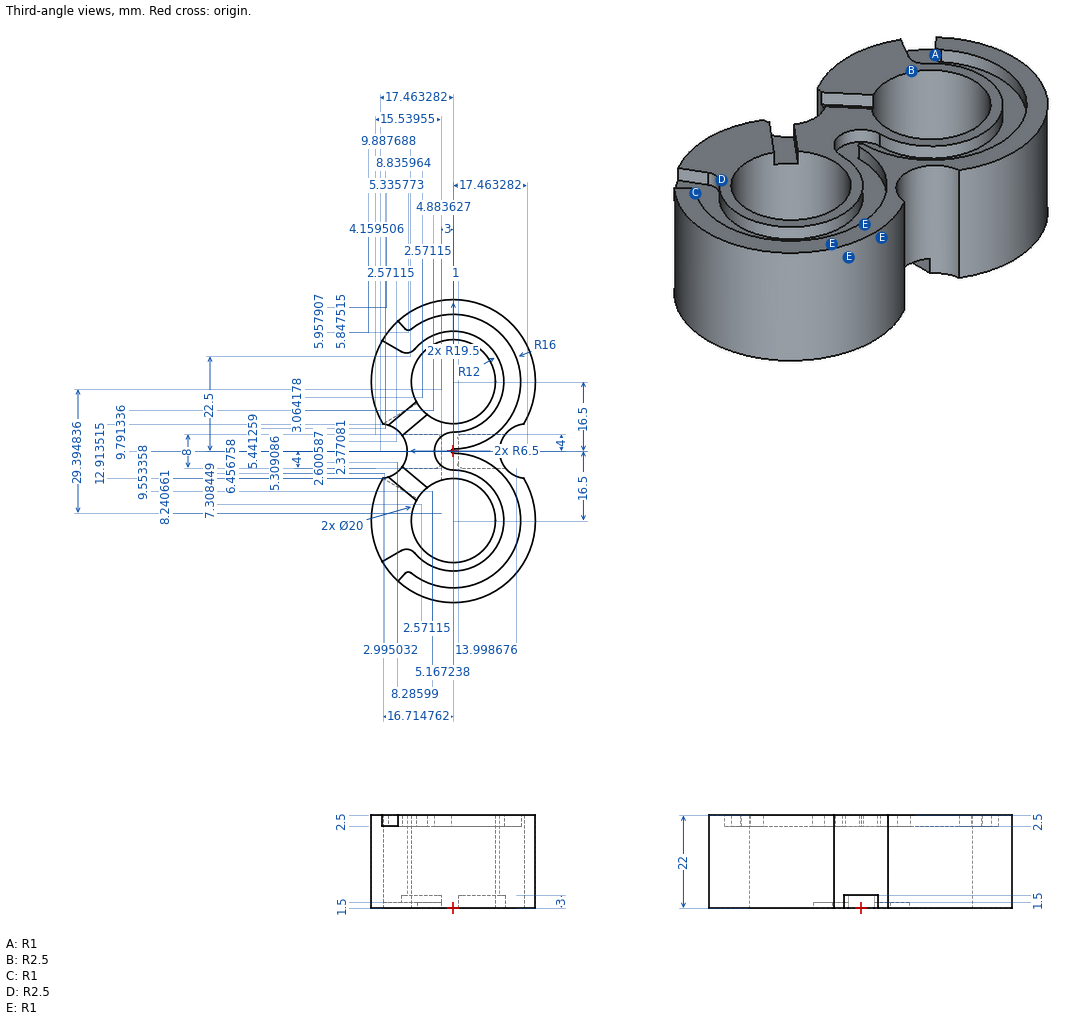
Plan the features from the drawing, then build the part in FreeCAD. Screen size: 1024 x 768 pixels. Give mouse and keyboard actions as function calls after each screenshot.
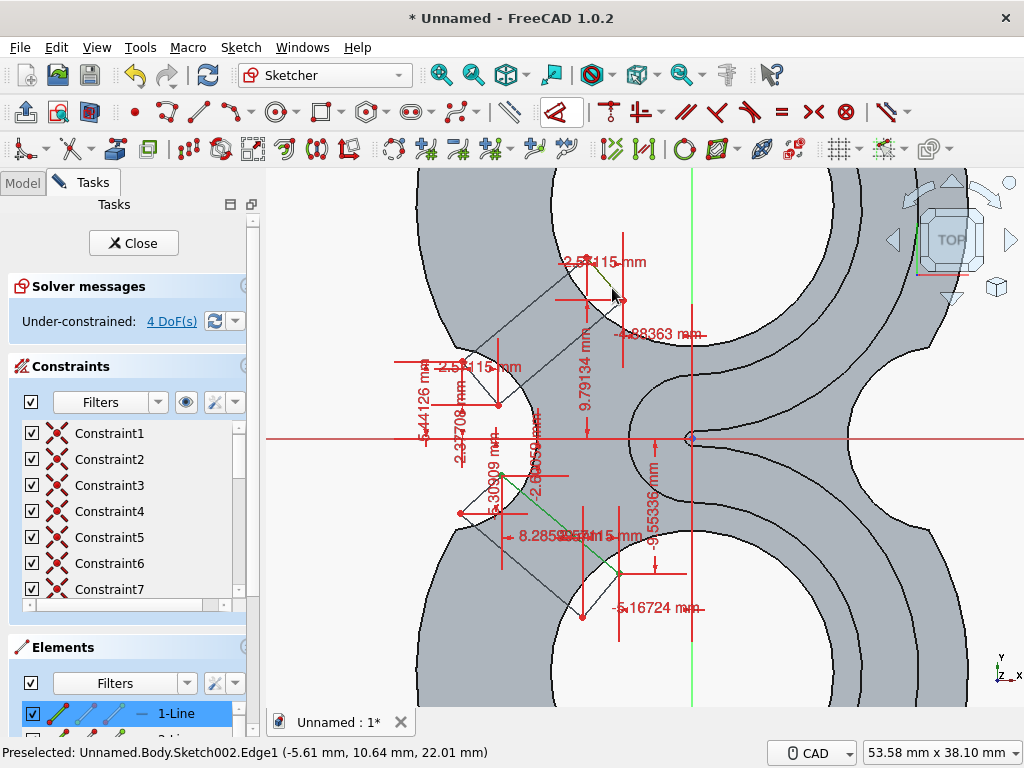
key(i)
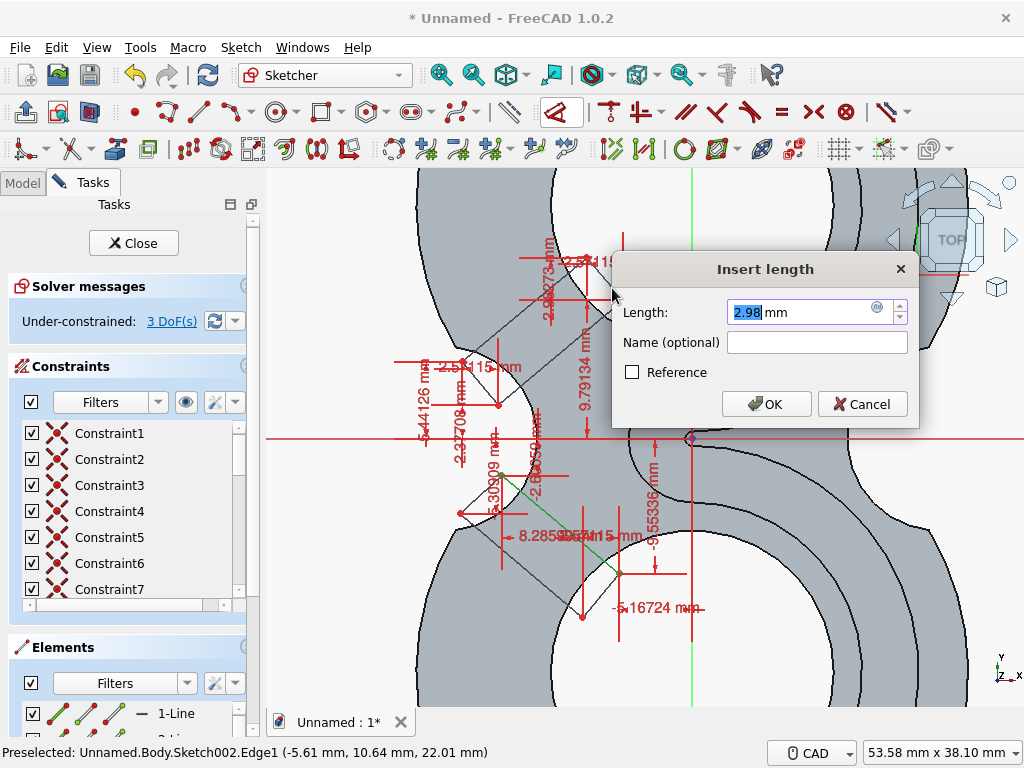
text(3.064178)
key(Return)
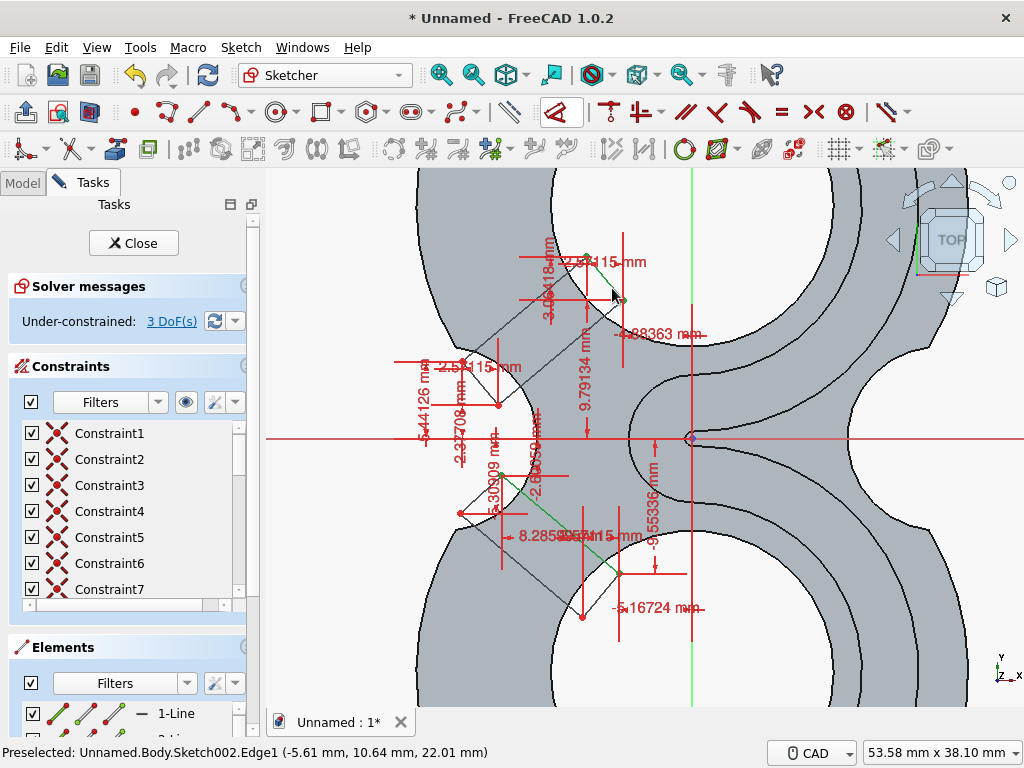
click(499, 330)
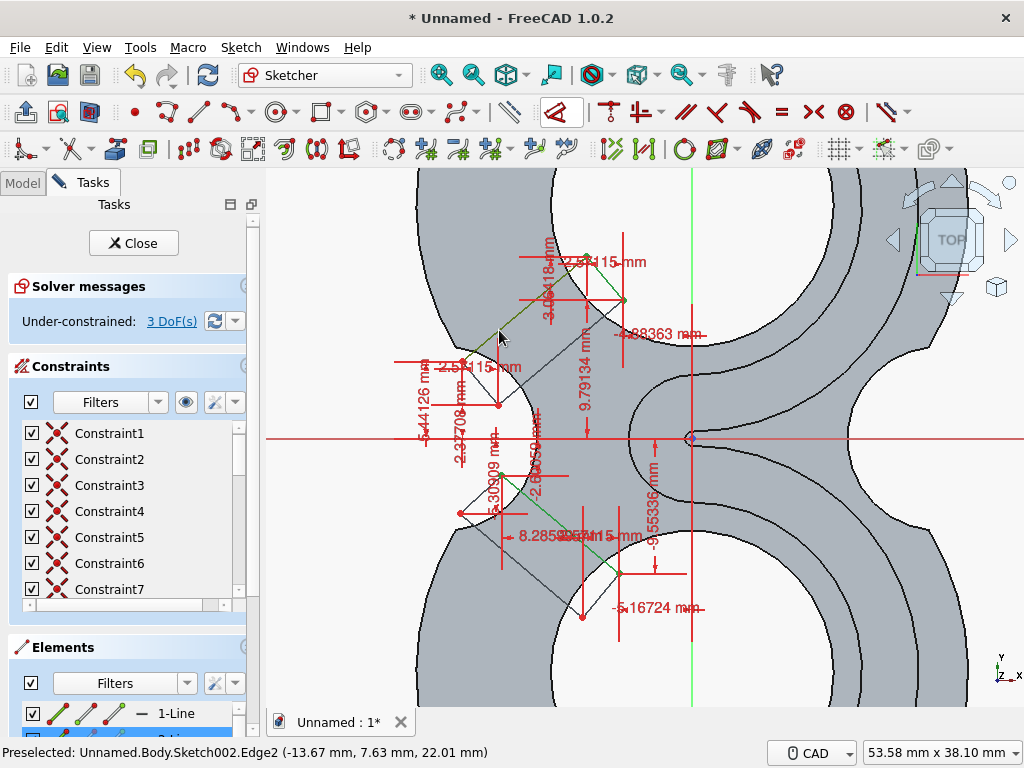
key(l)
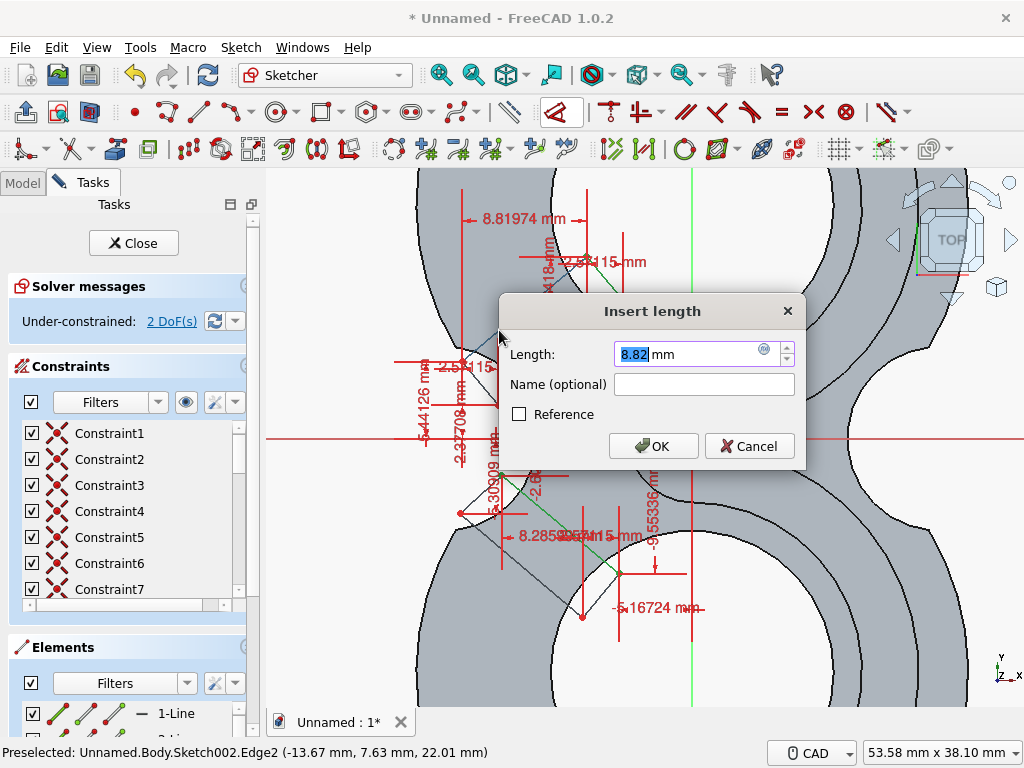
text(8.835964)
key(Return)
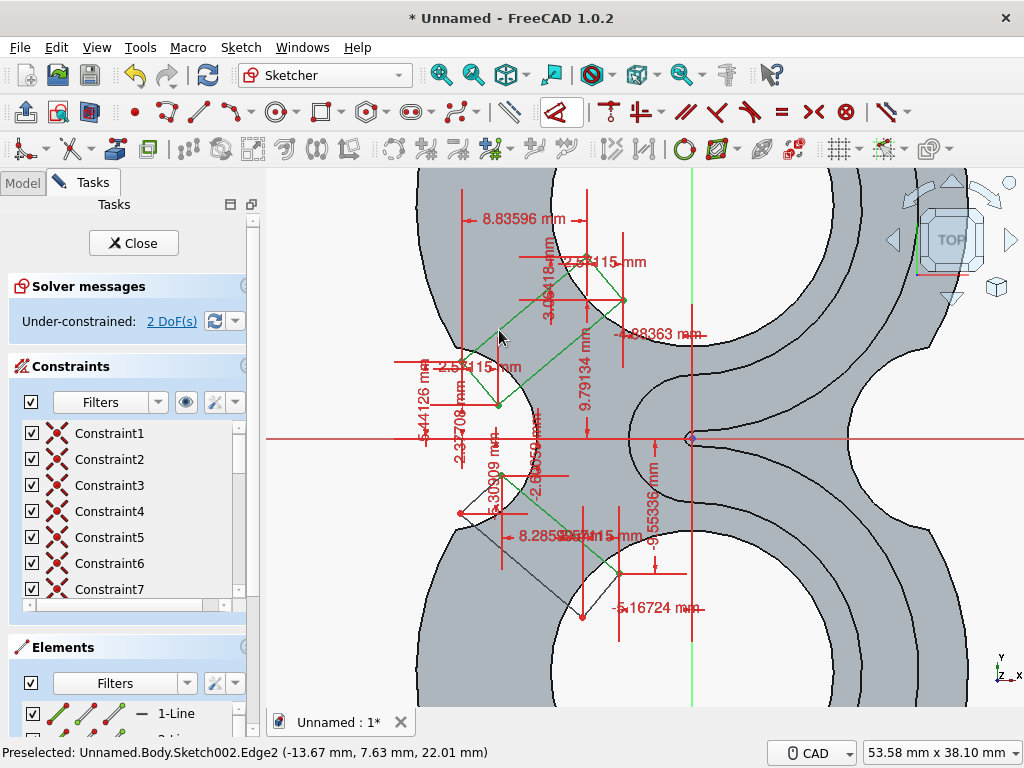
click(473, 502)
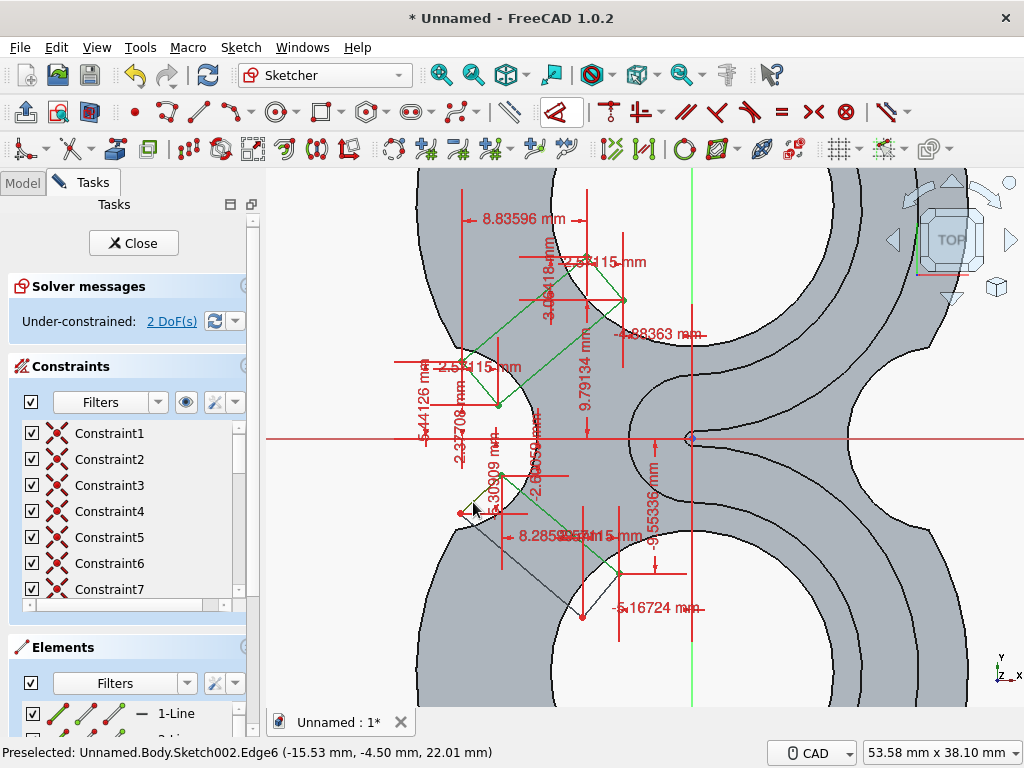
key(l)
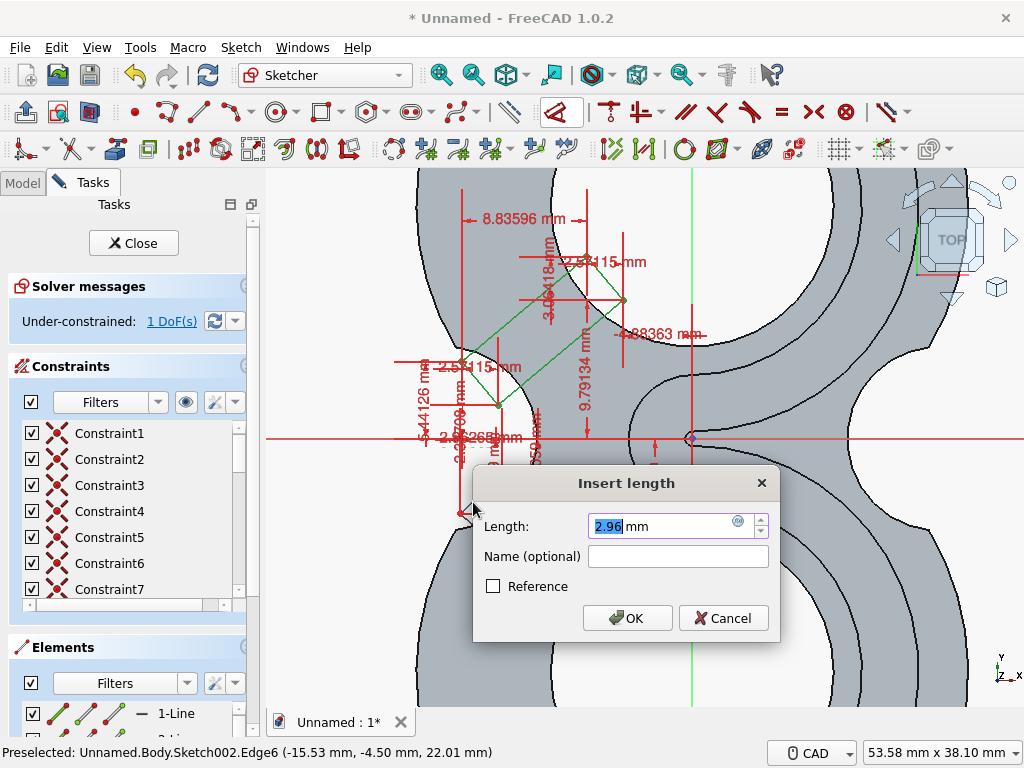
text(2.995032)
key(Return)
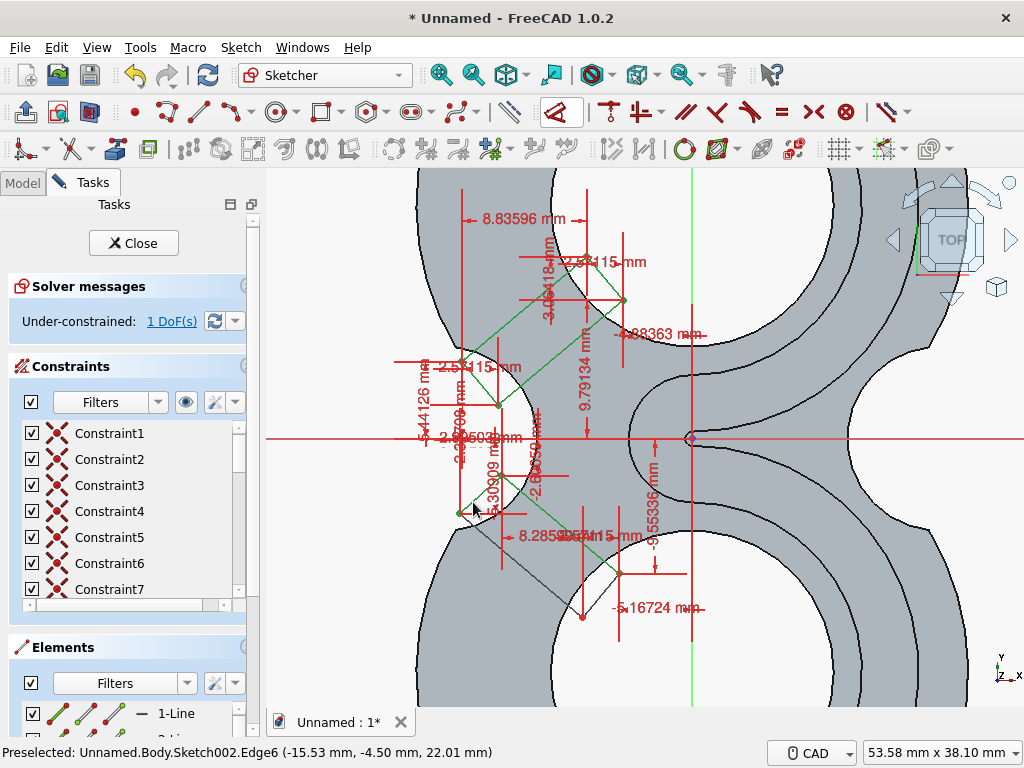
click(497, 545)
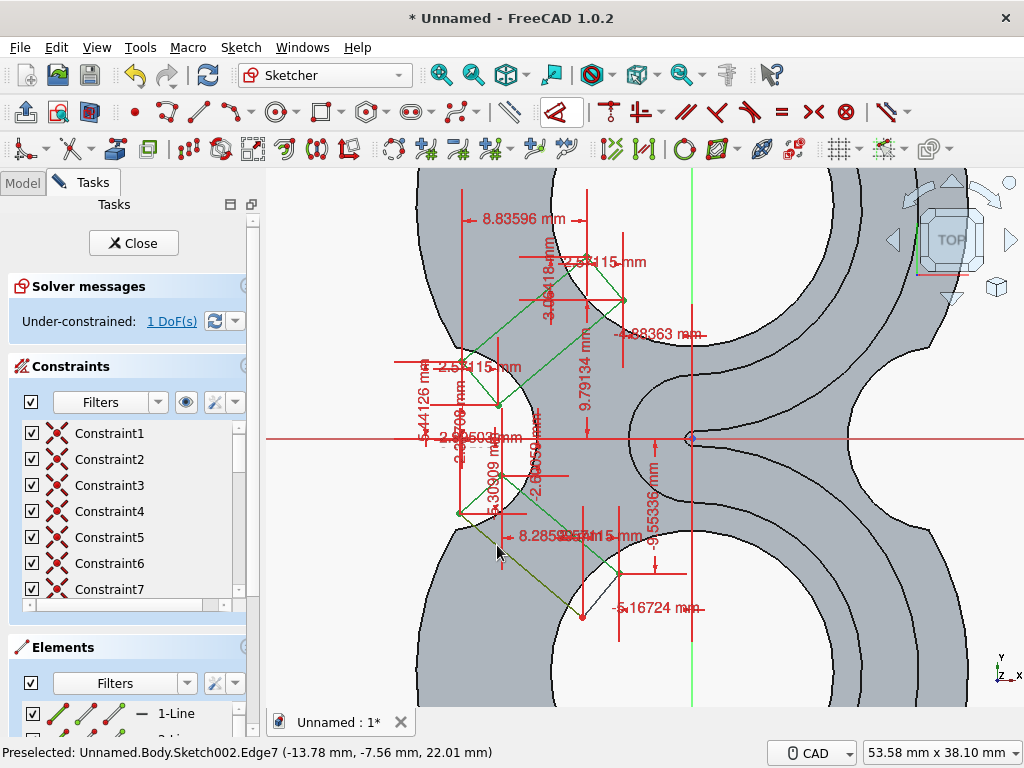
click(578, 112)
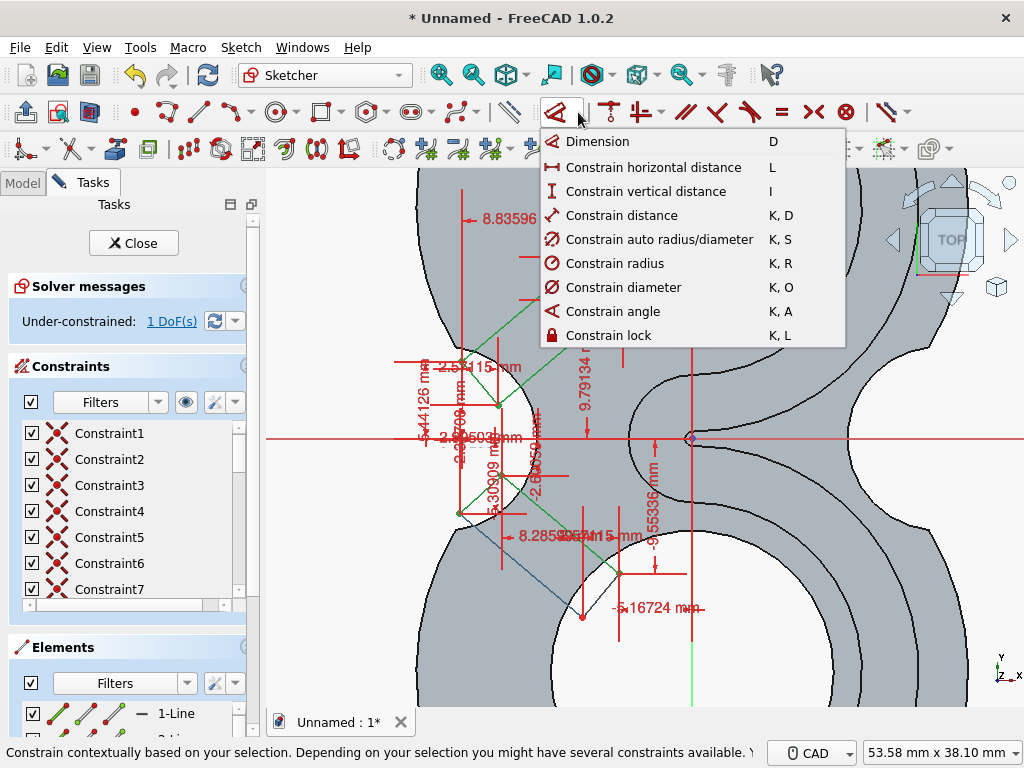
click(693, 191)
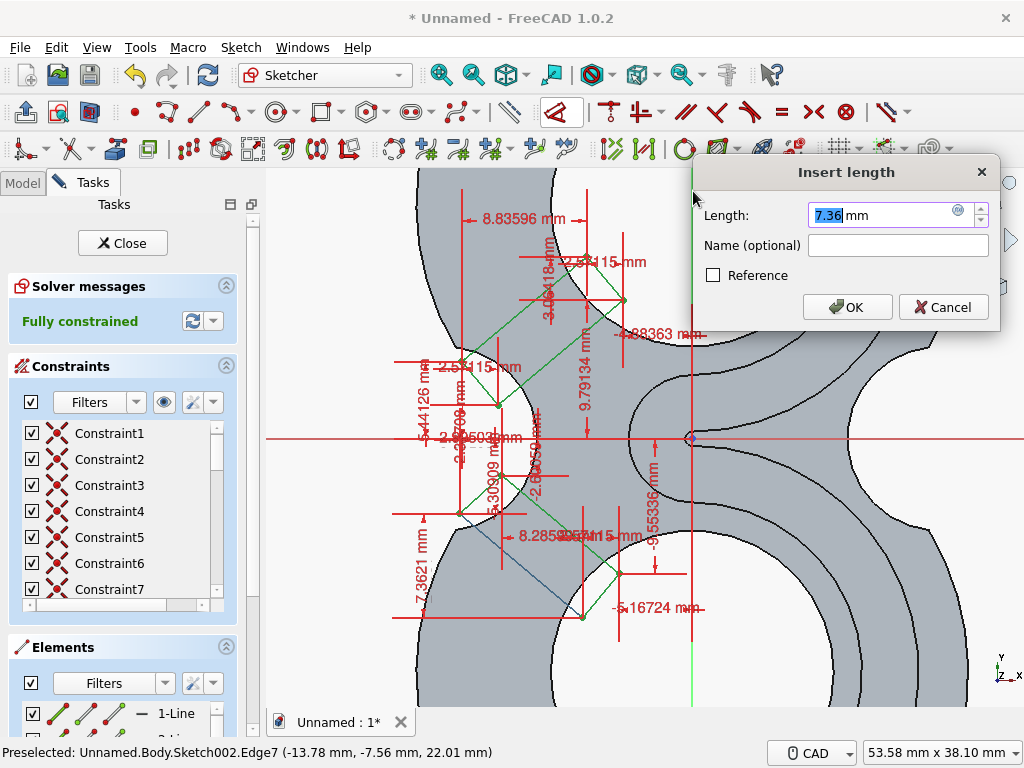
text(7.308449)
key(Return)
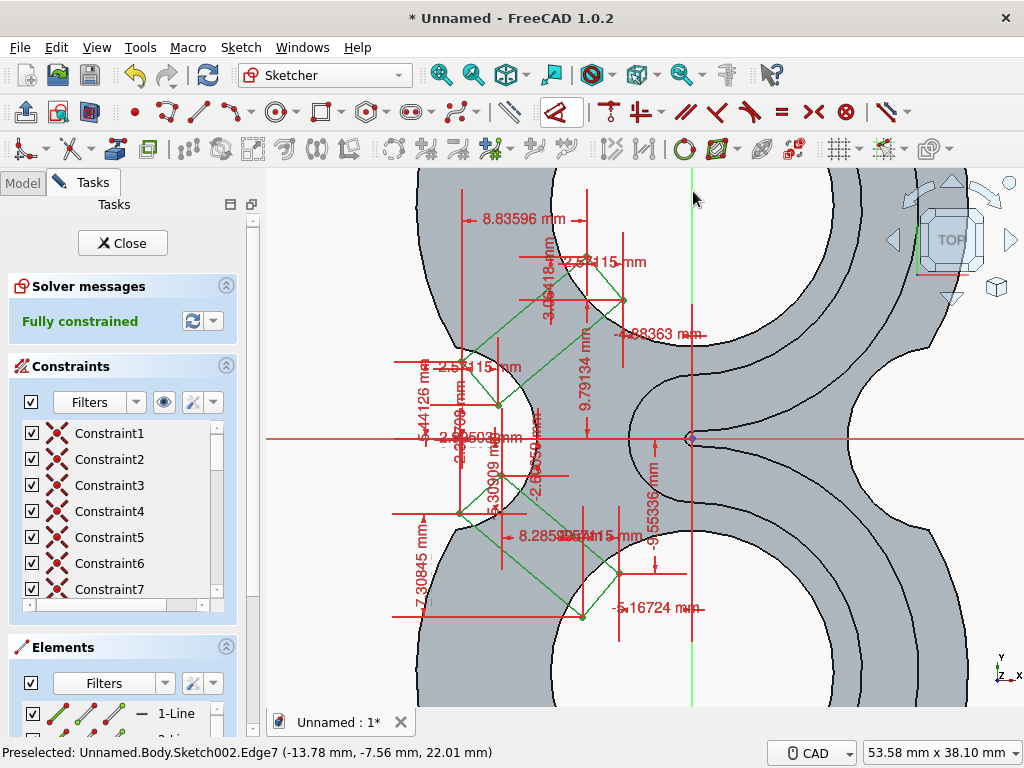
click(123, 243)